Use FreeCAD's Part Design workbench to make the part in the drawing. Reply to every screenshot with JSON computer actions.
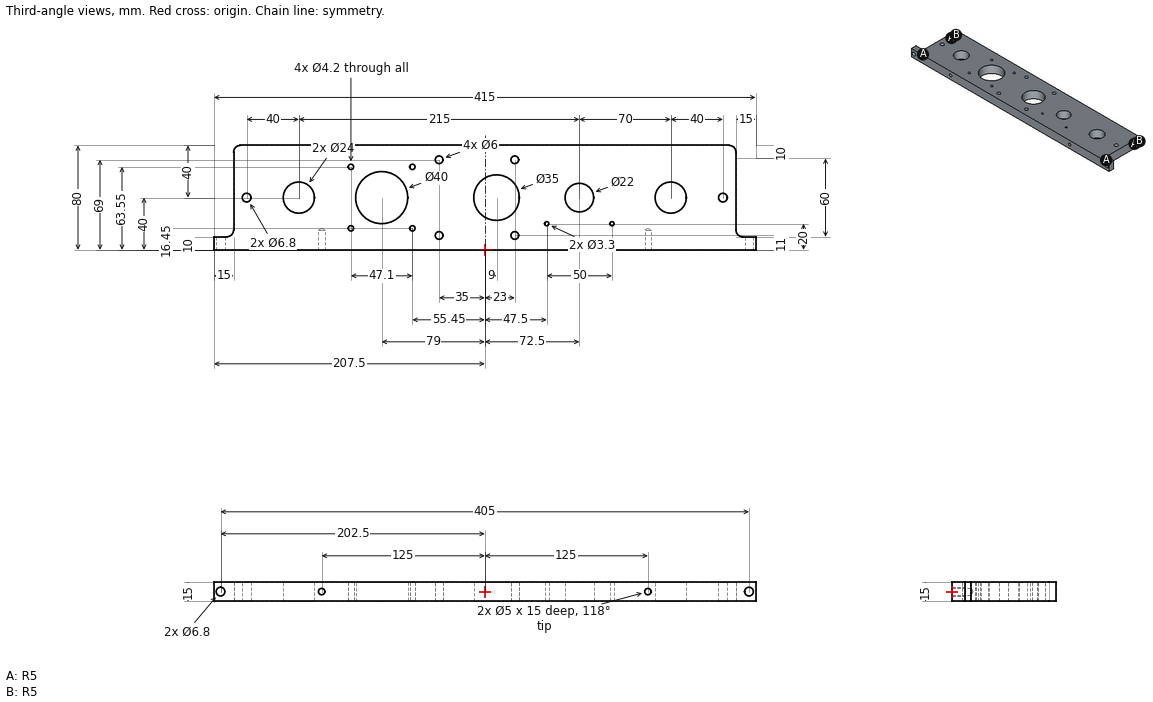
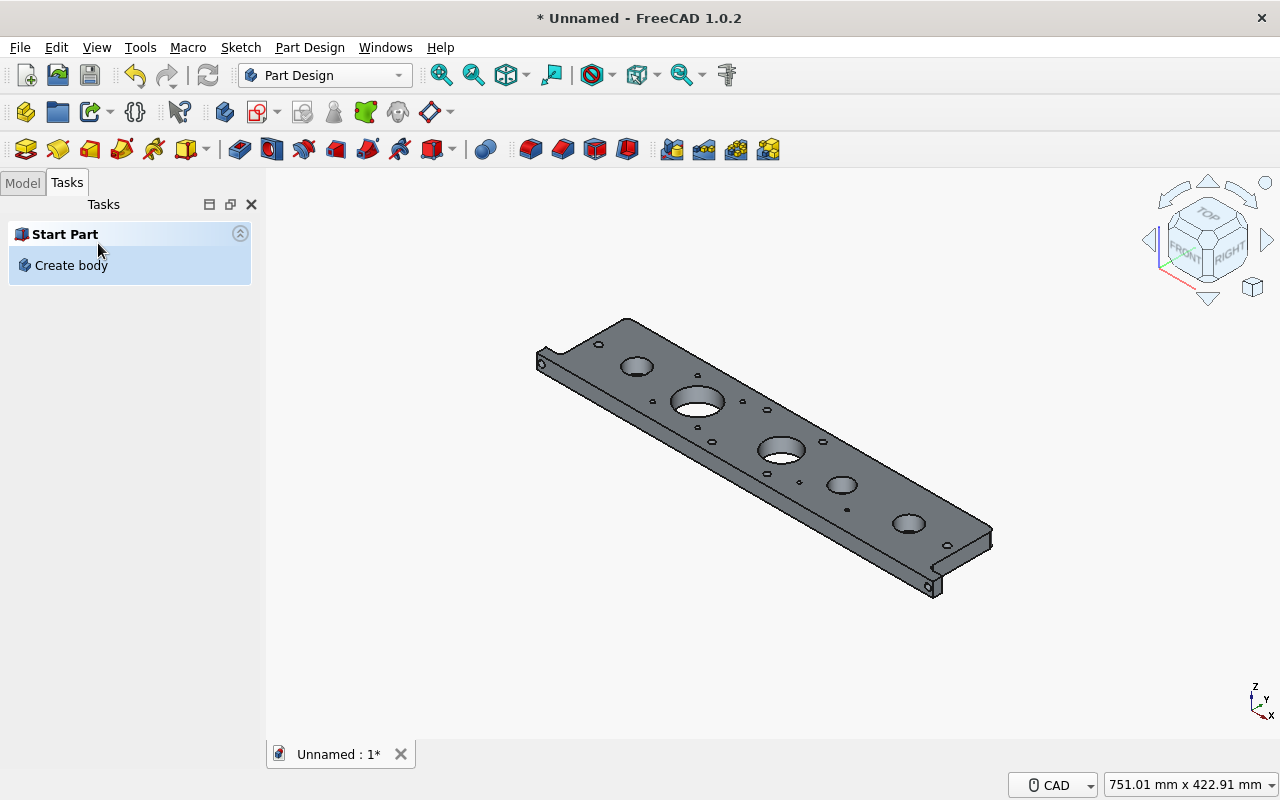
{"action": "key", "text": "1"}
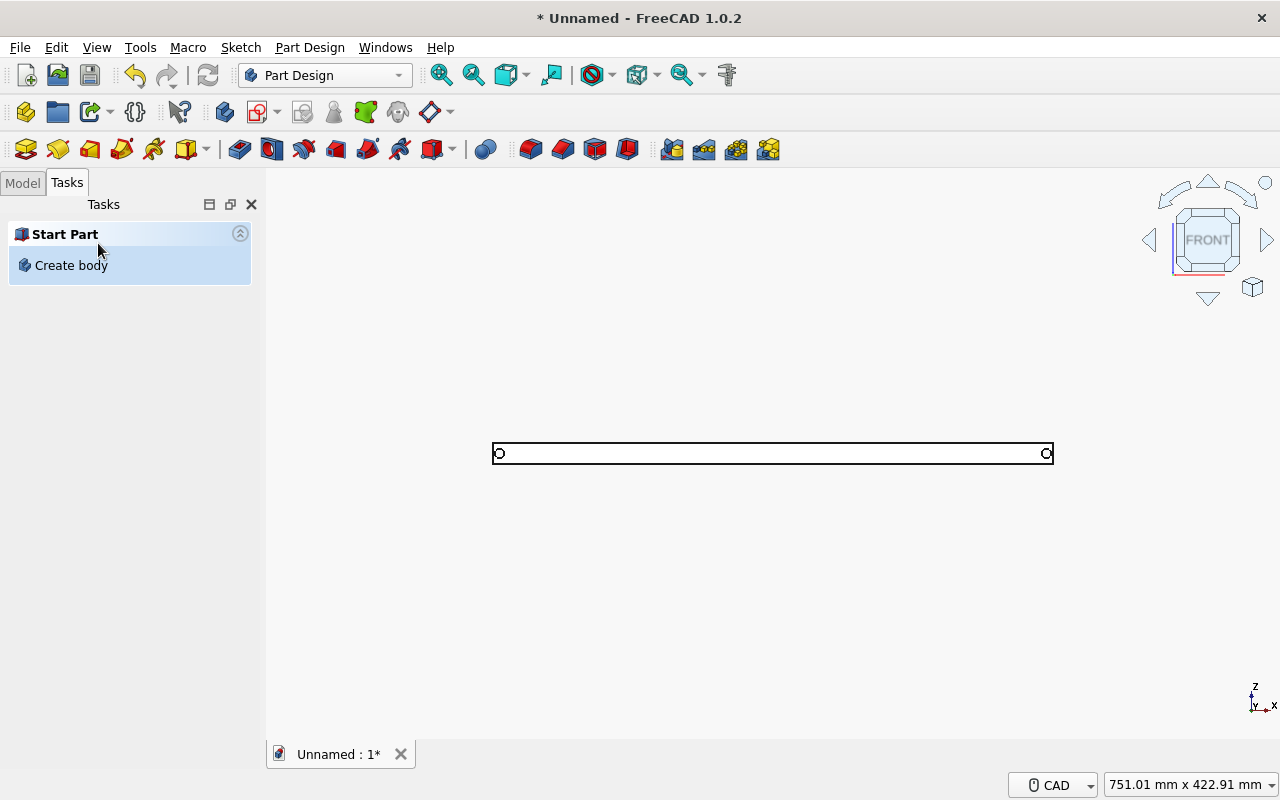
{"action": "left_click", "coordinate": [1013, 452]}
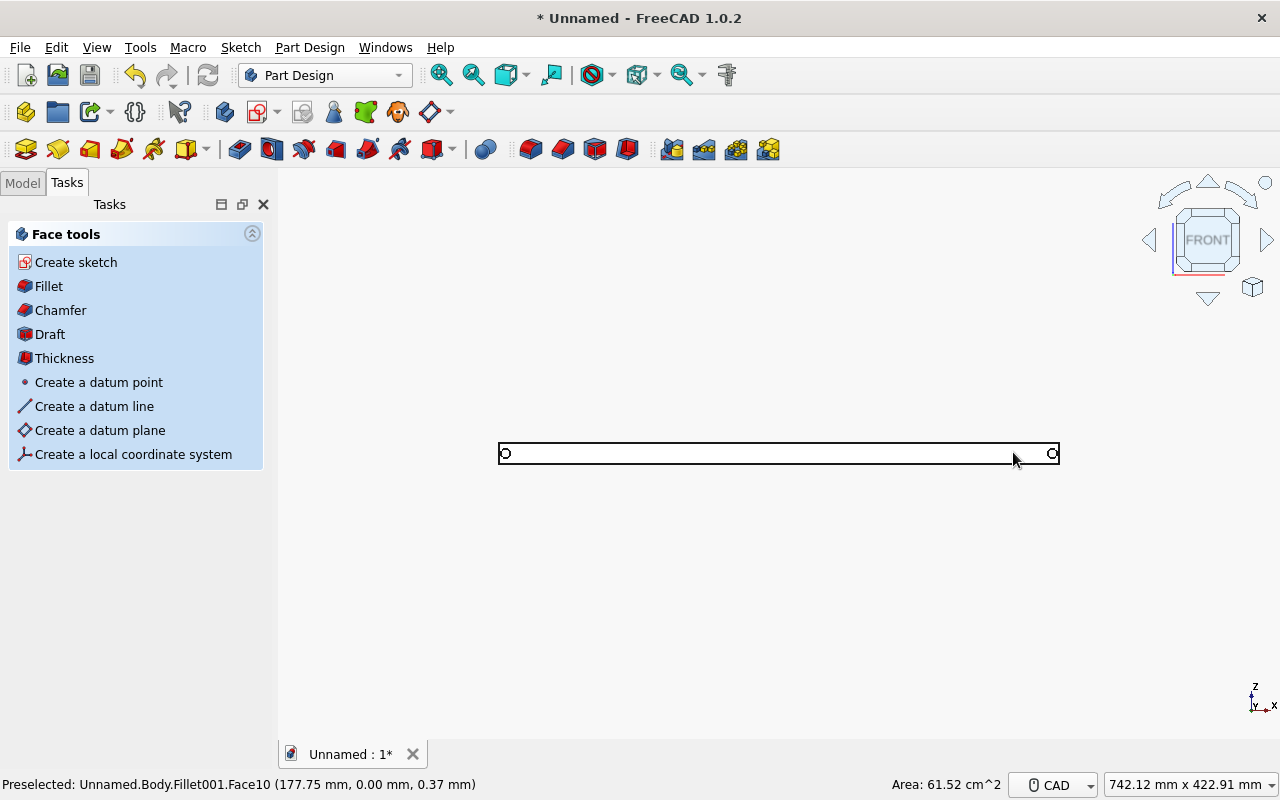
{"action": "left_click", "coordinate": [258, 112]}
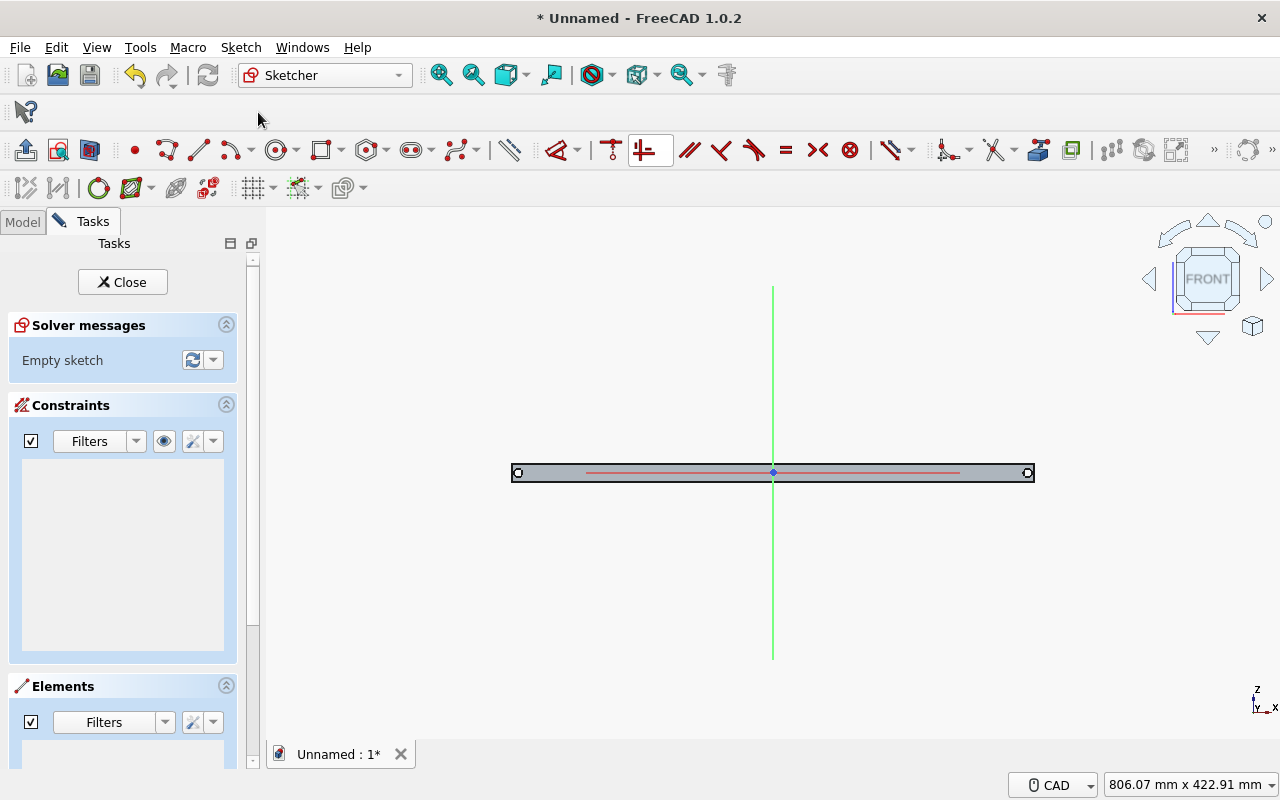
{"action": "scroll", "coordinate": [856, 473], "scroll_direction": "up", "scroll_amount": 3}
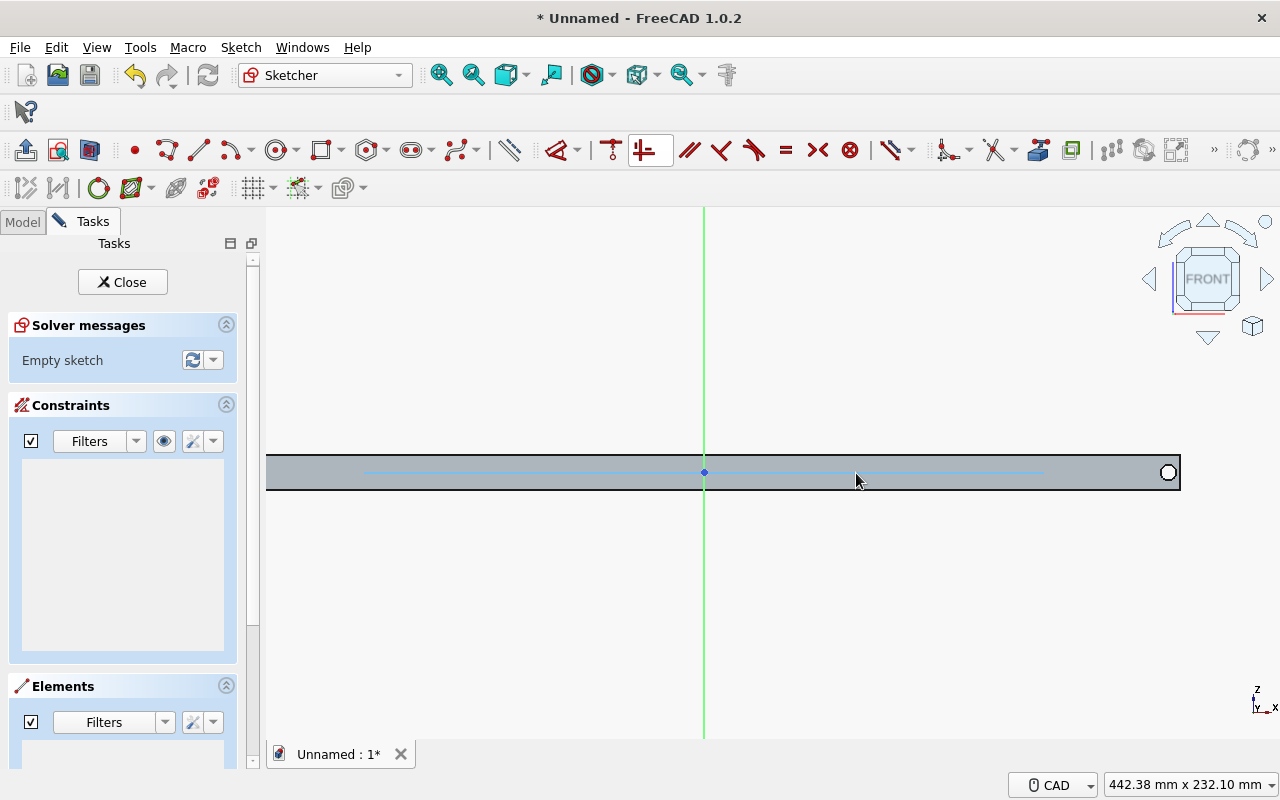
{"action": "left_click", "coordinate": [276, 150]}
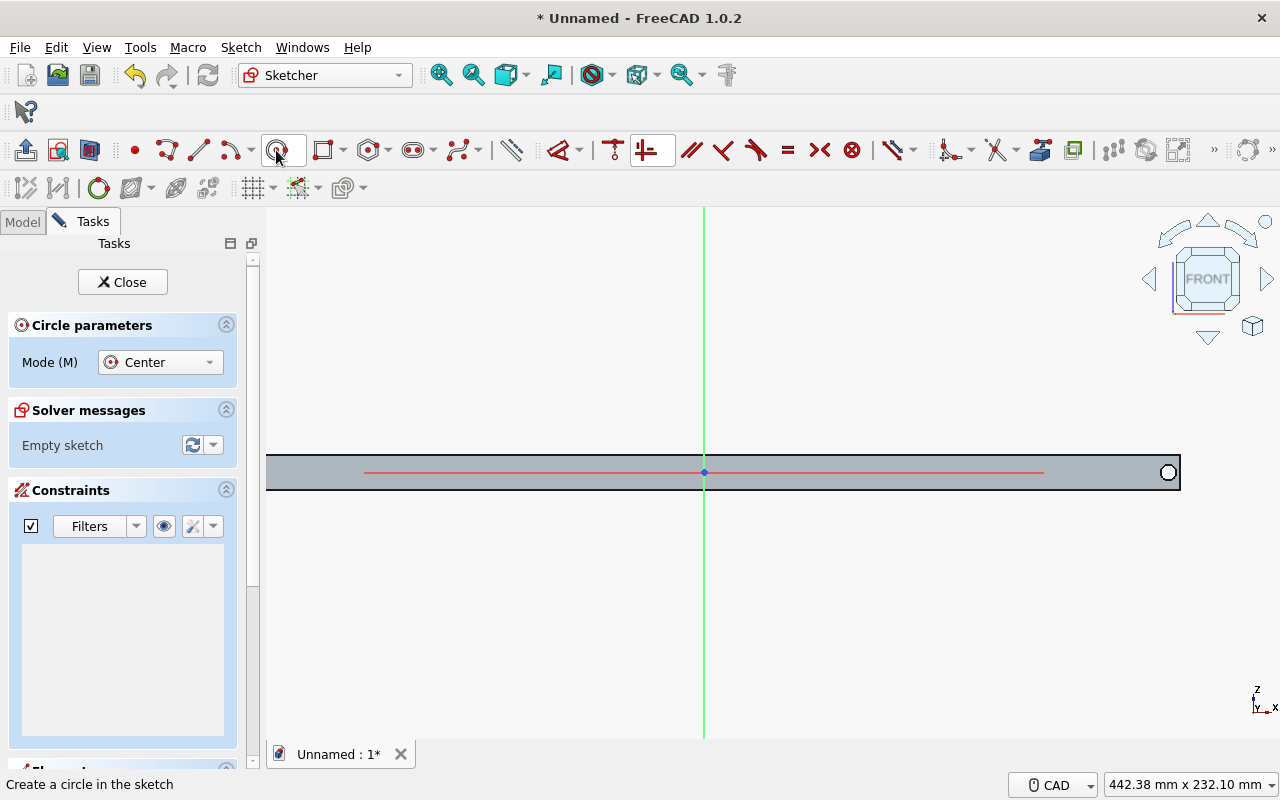
{"action": "scroll", "coordinate": [991, 473], "scroll_direction": "up", "scroll_amount": 7}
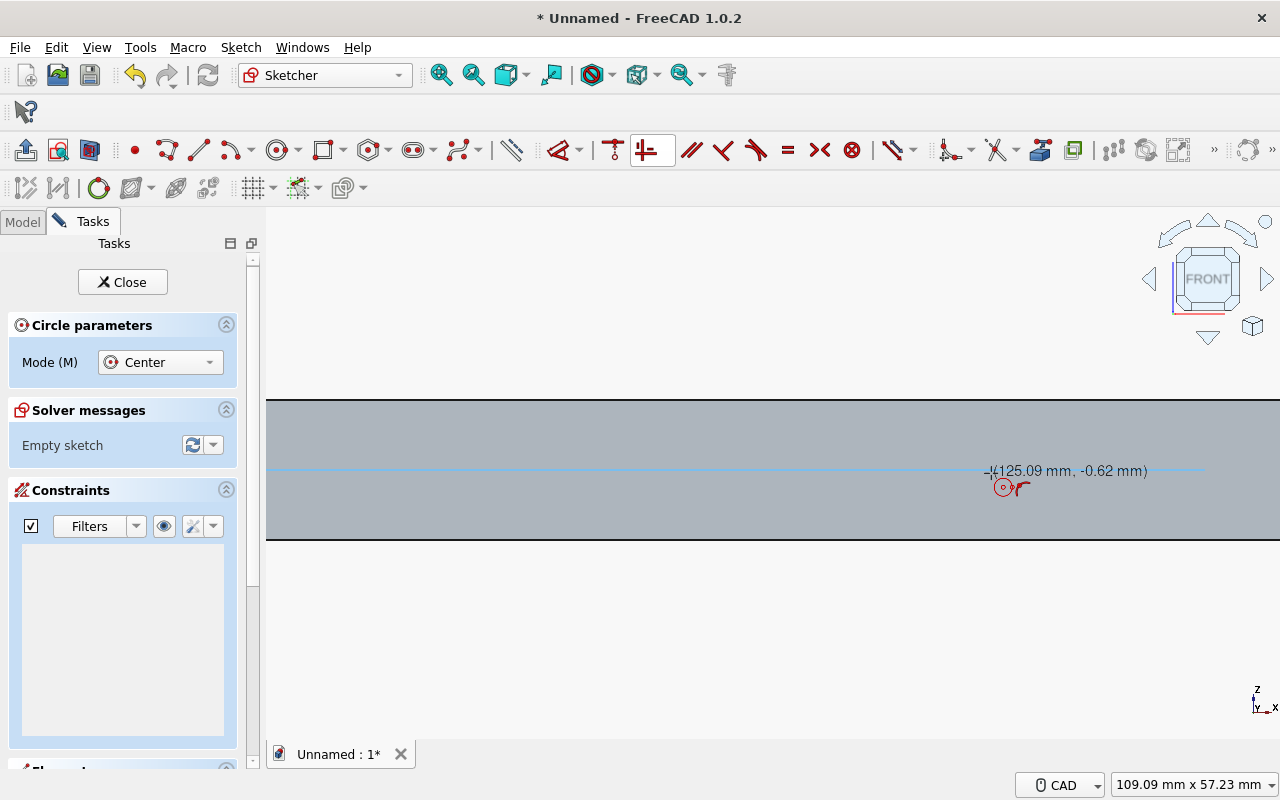
{"action": "scroll", "coordinate": [992, 474], "scroll_direction": "down", "scroll_amount": 7}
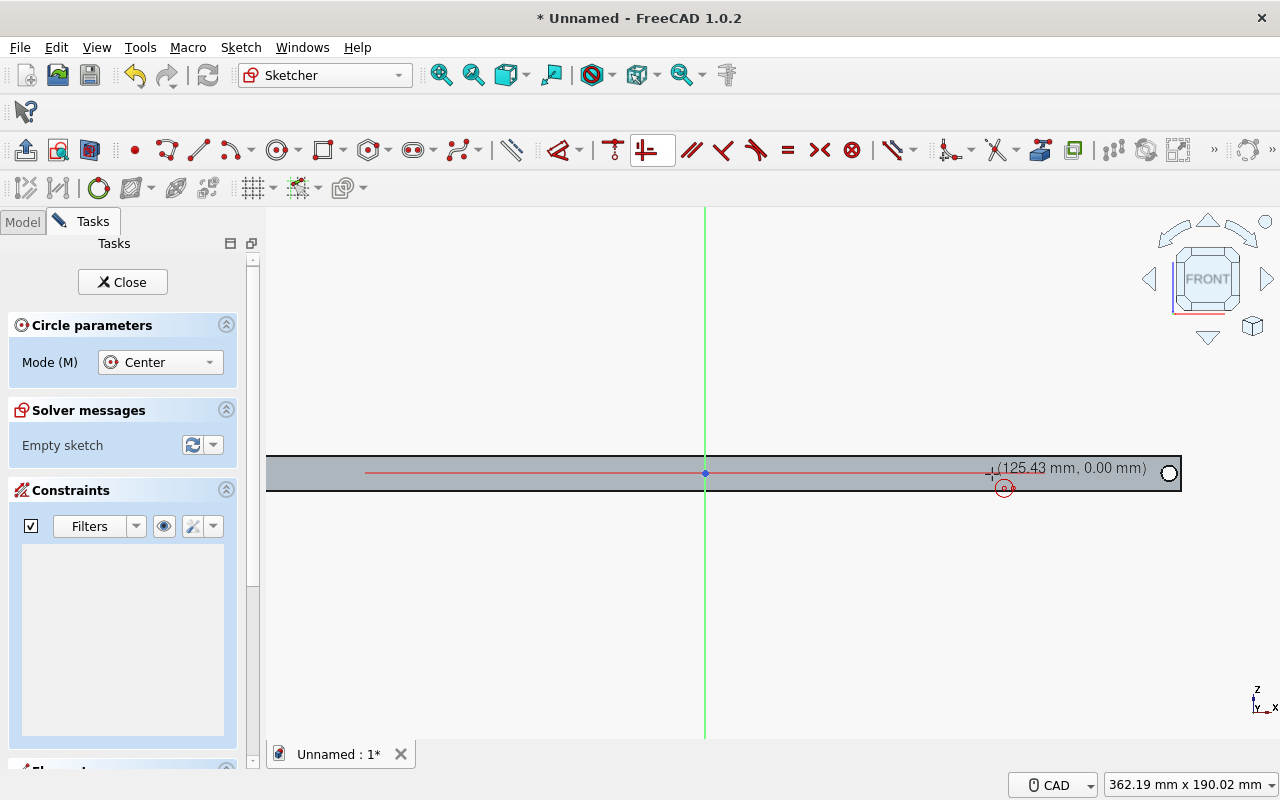
{"action": "left_click", "coordinate": [992, 473]}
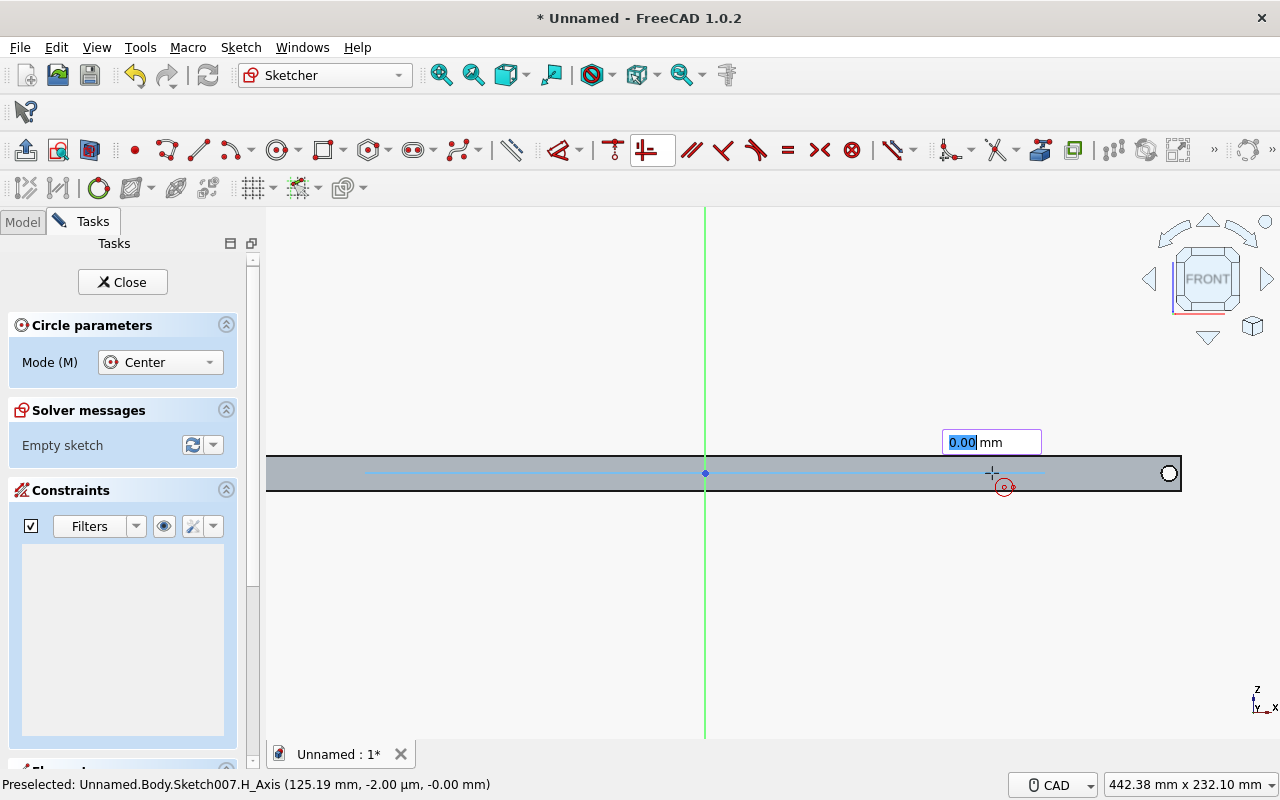
{"action": "scroll", "coordinate": [990, 479], "scroll_direction": "up", "scroll_amount": 6}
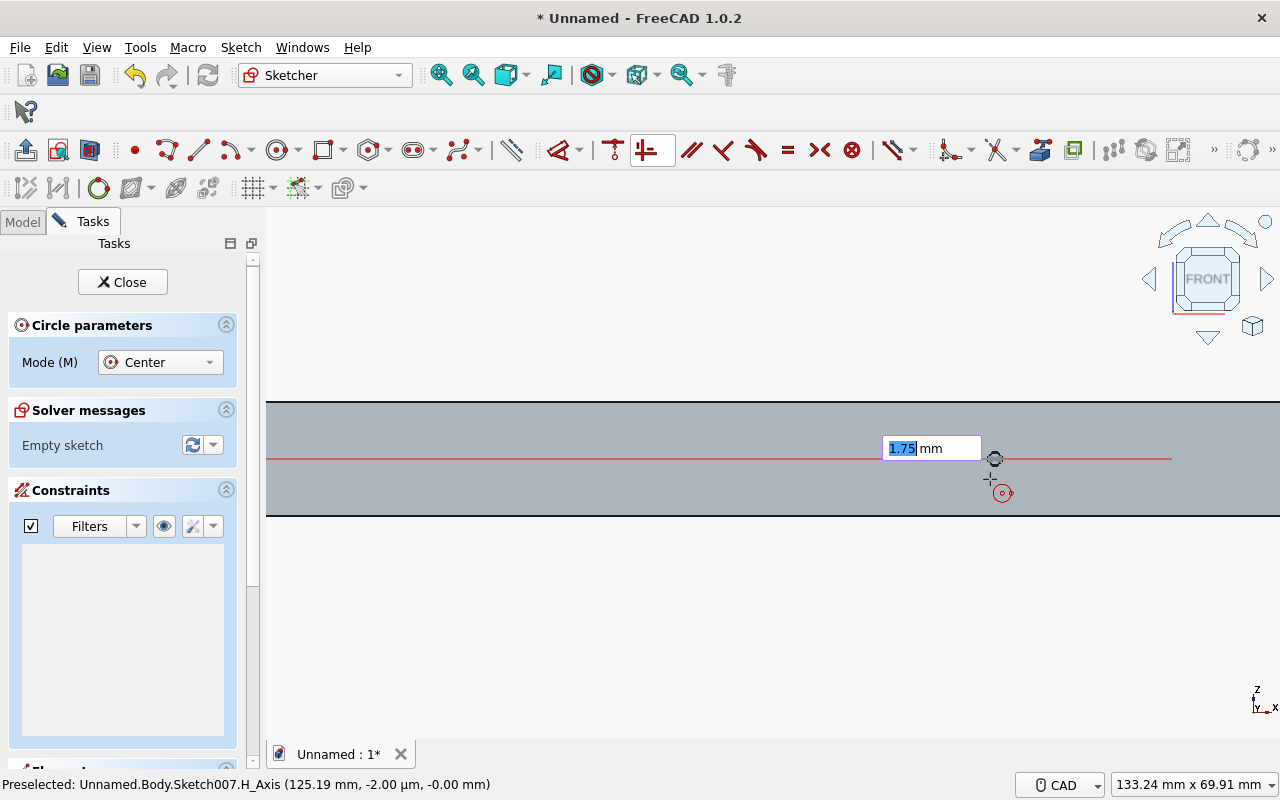
{"action": "left_click", "coordinate": [987, 477]}